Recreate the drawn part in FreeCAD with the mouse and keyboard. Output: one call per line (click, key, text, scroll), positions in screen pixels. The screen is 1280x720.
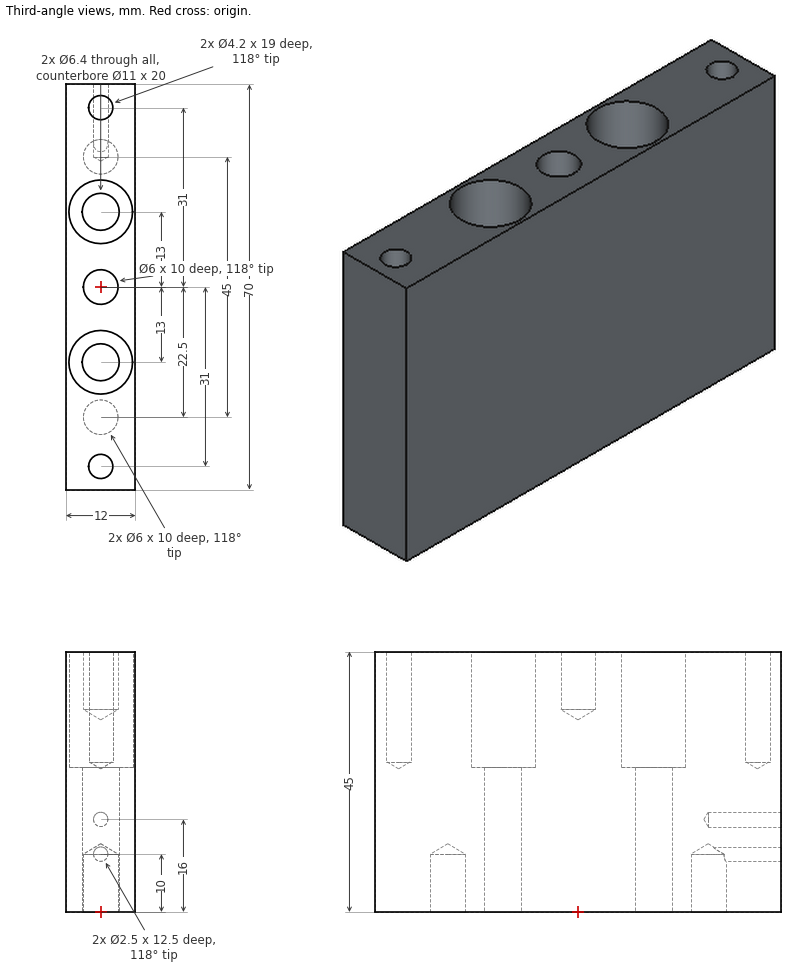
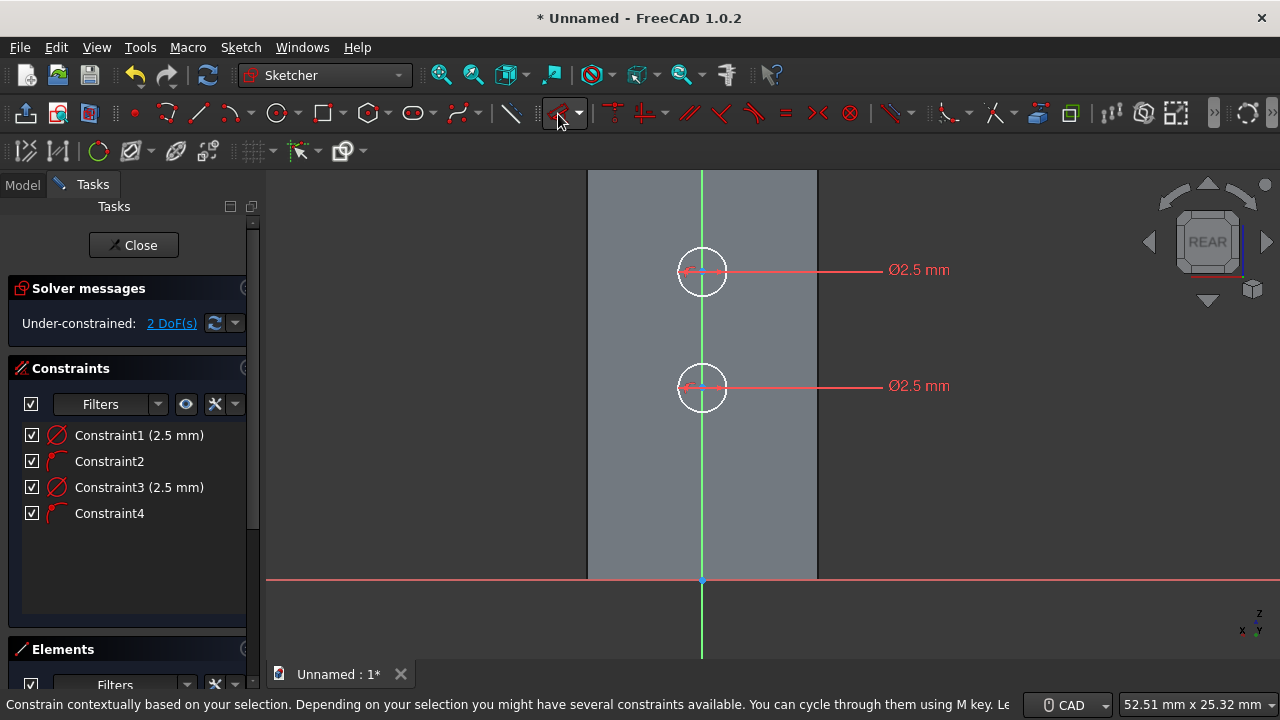
click(702, 388)
click(736, 484)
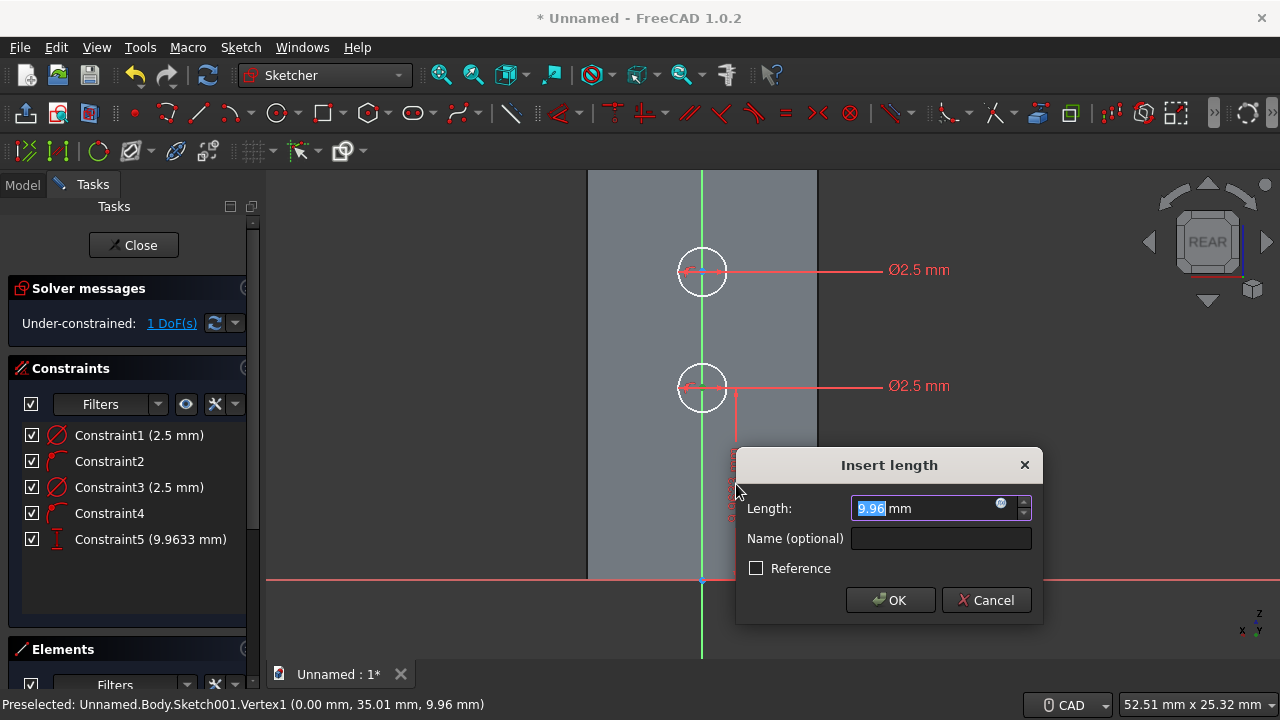
text(10)
key(Return)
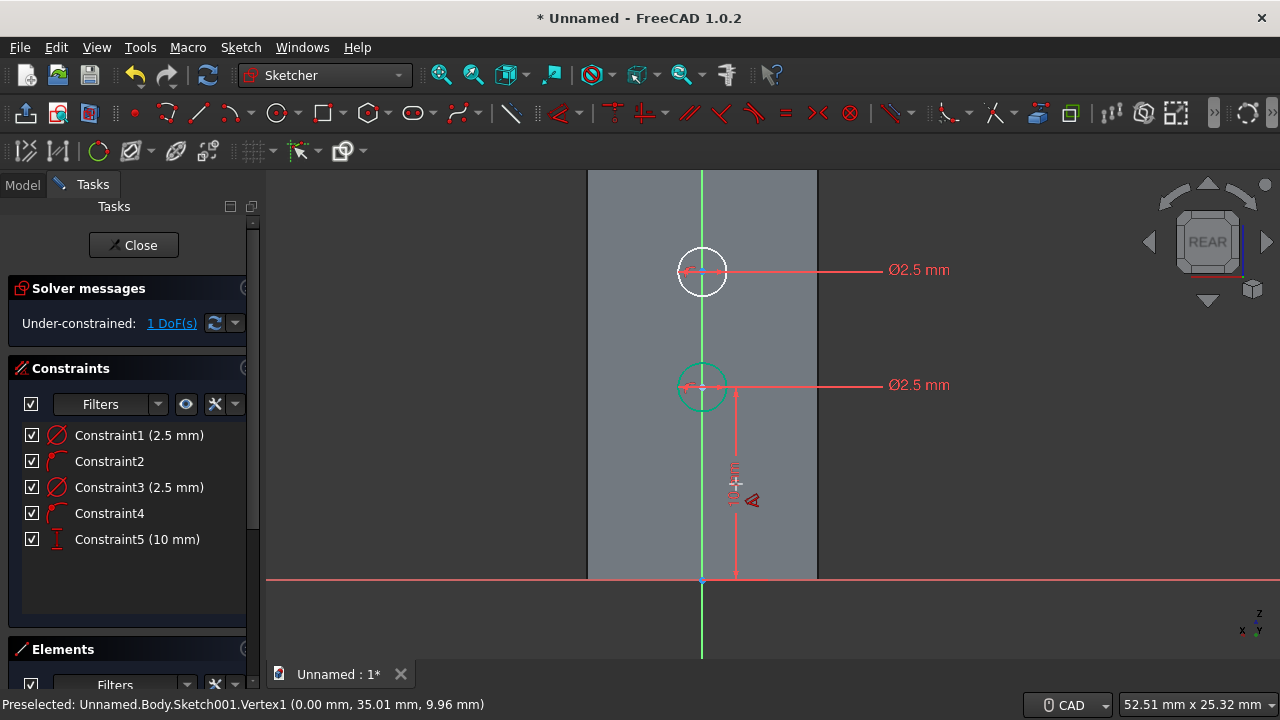
click(702, 272)
click(736, 426)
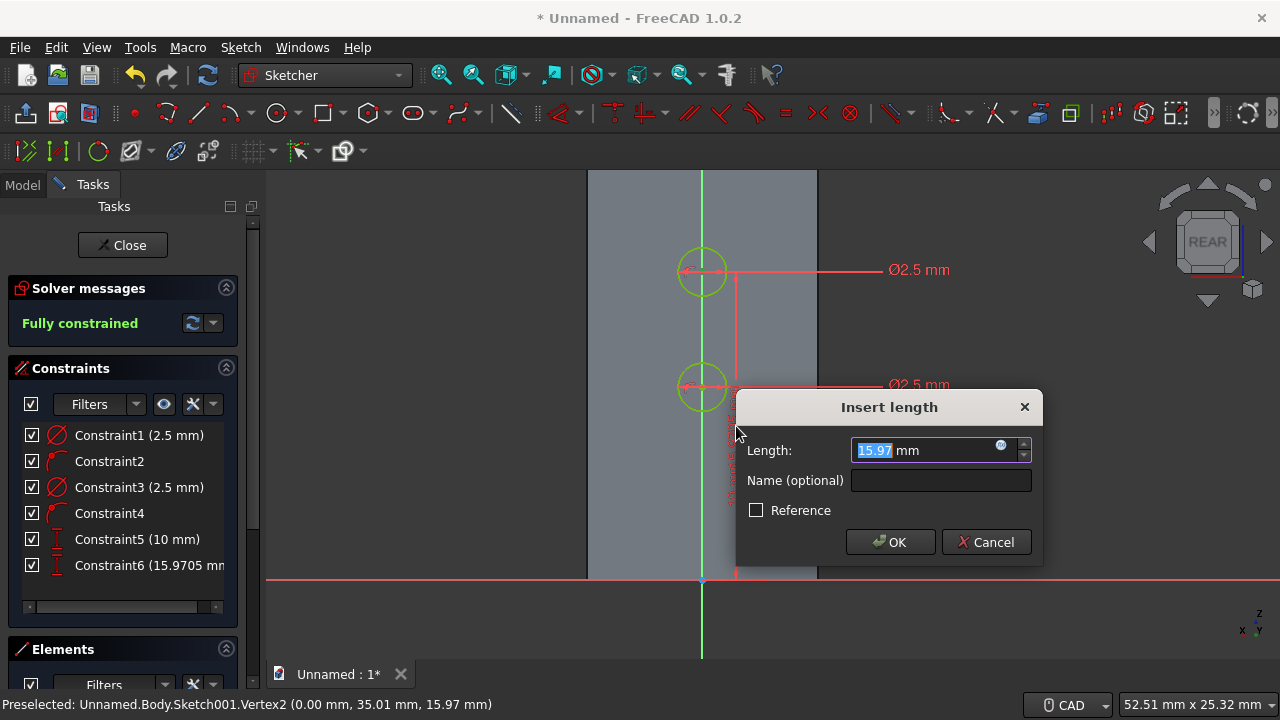
text(16)
key(Return)
key(Escape)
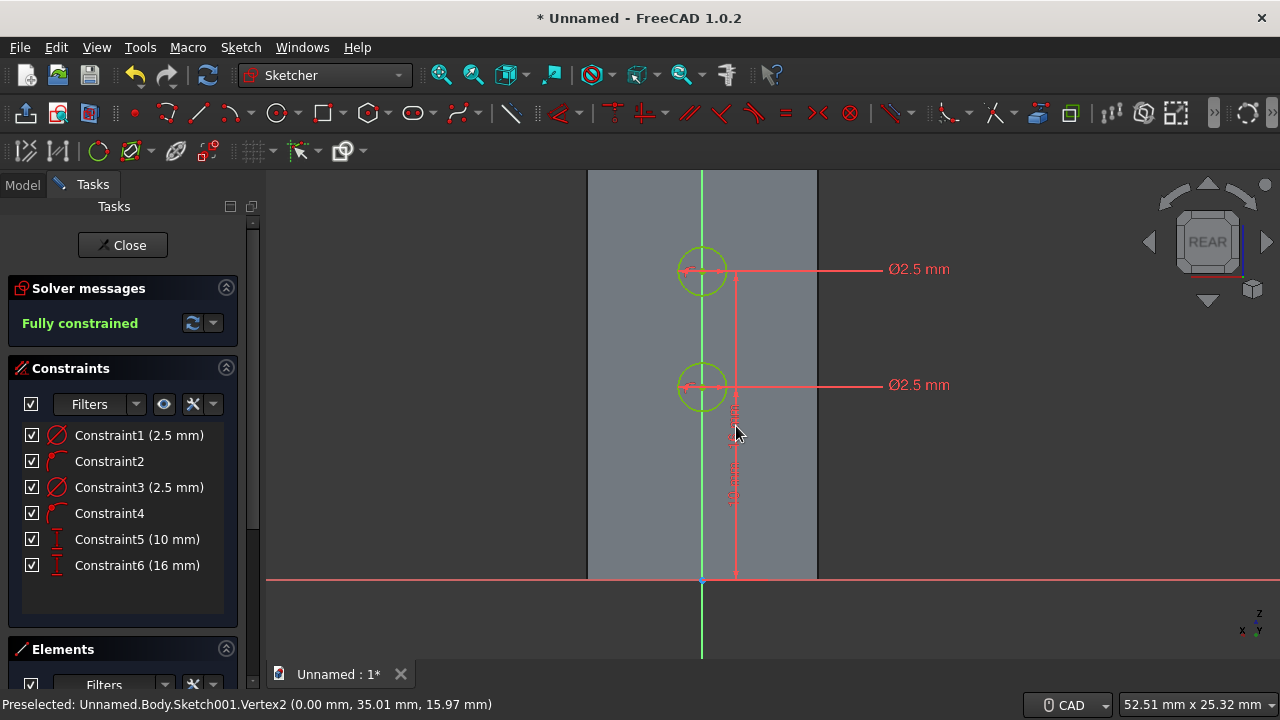
click(123, 245)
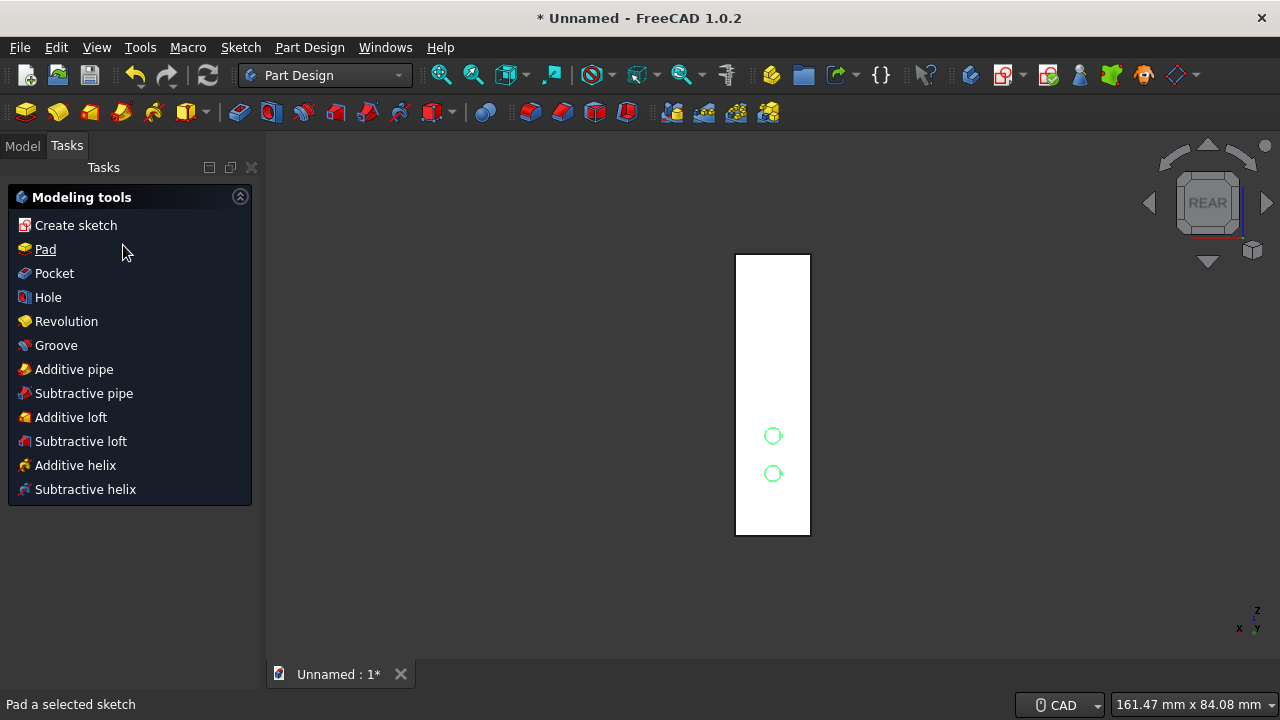
click(272, 112)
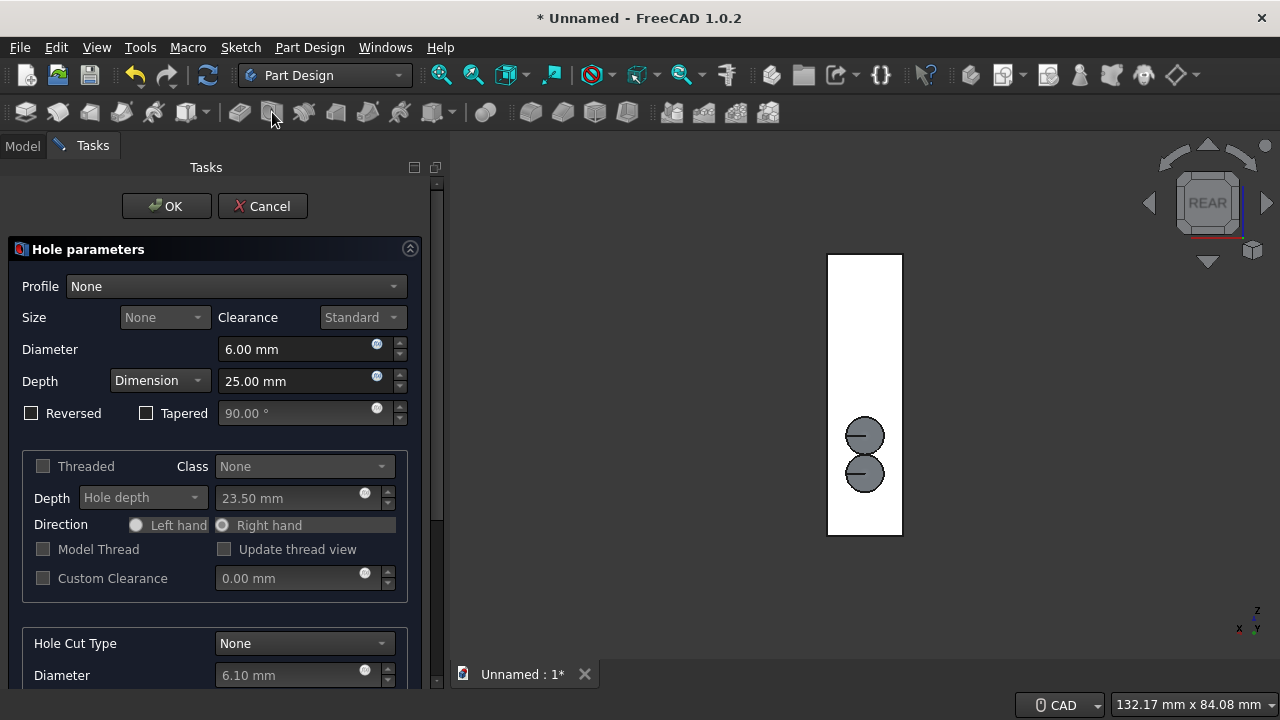
triple_click(305, 349)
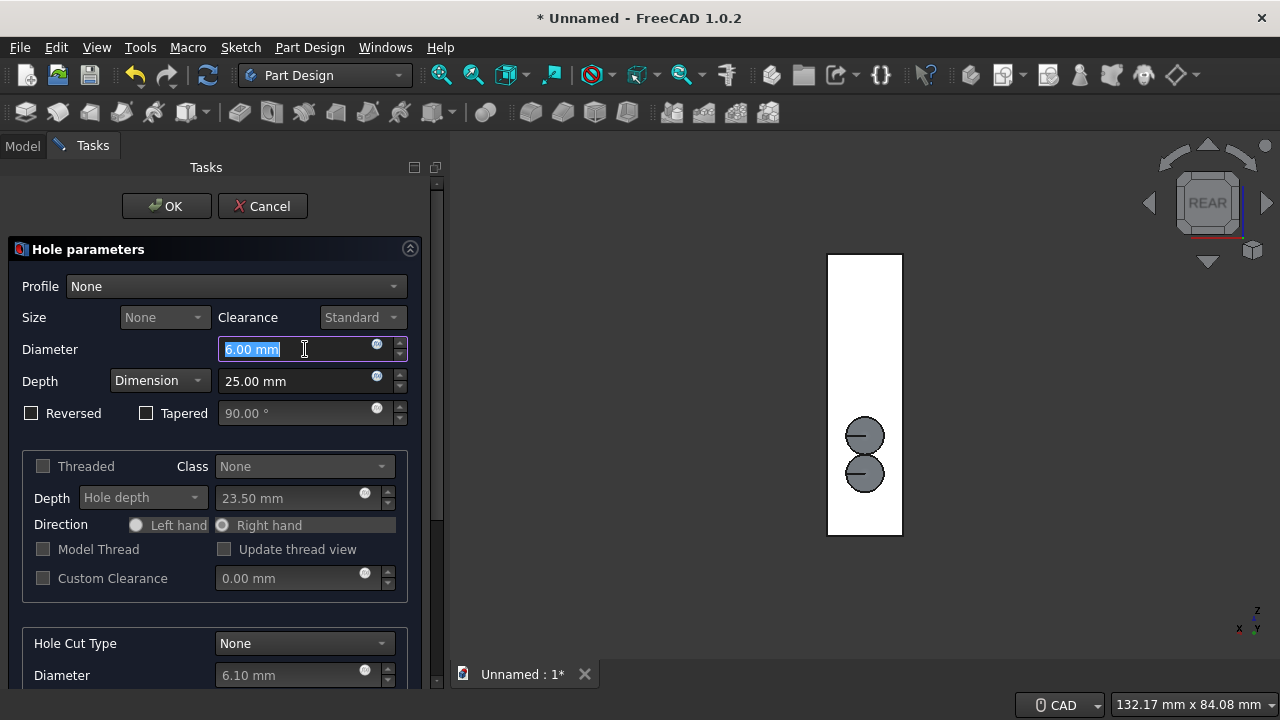
text(2.5)
key(Tab)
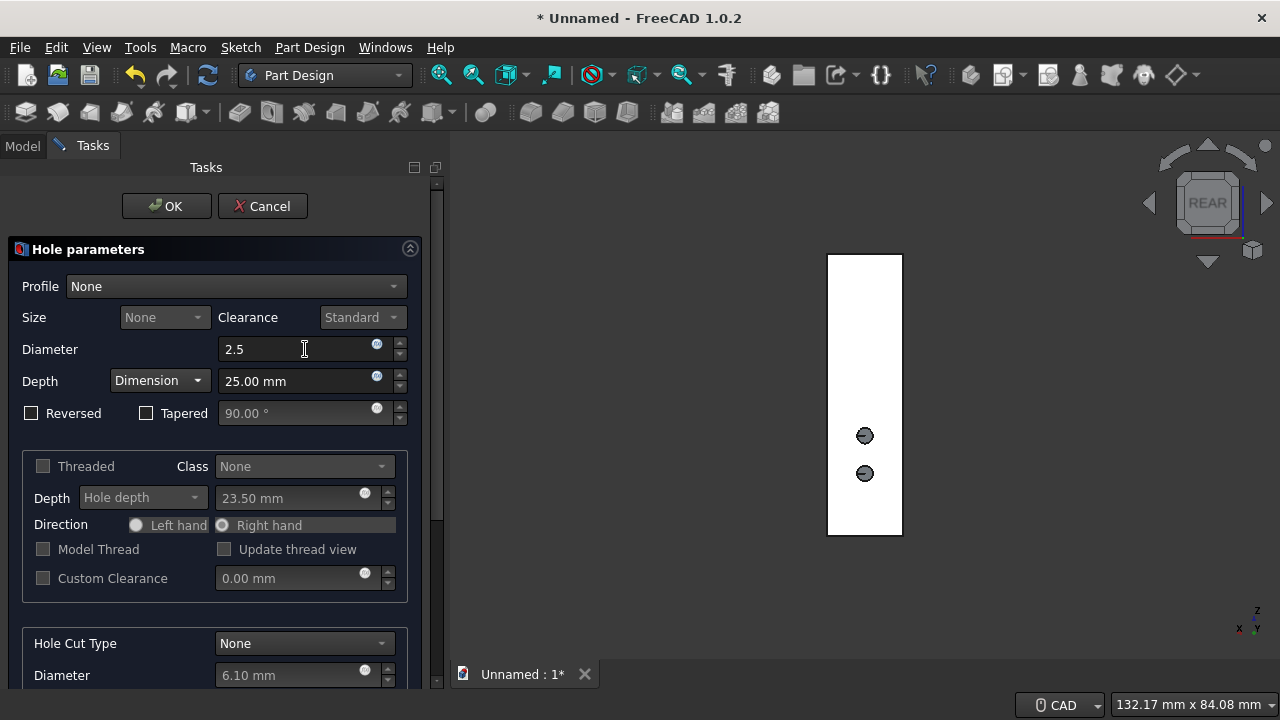
triple_click(305, 381)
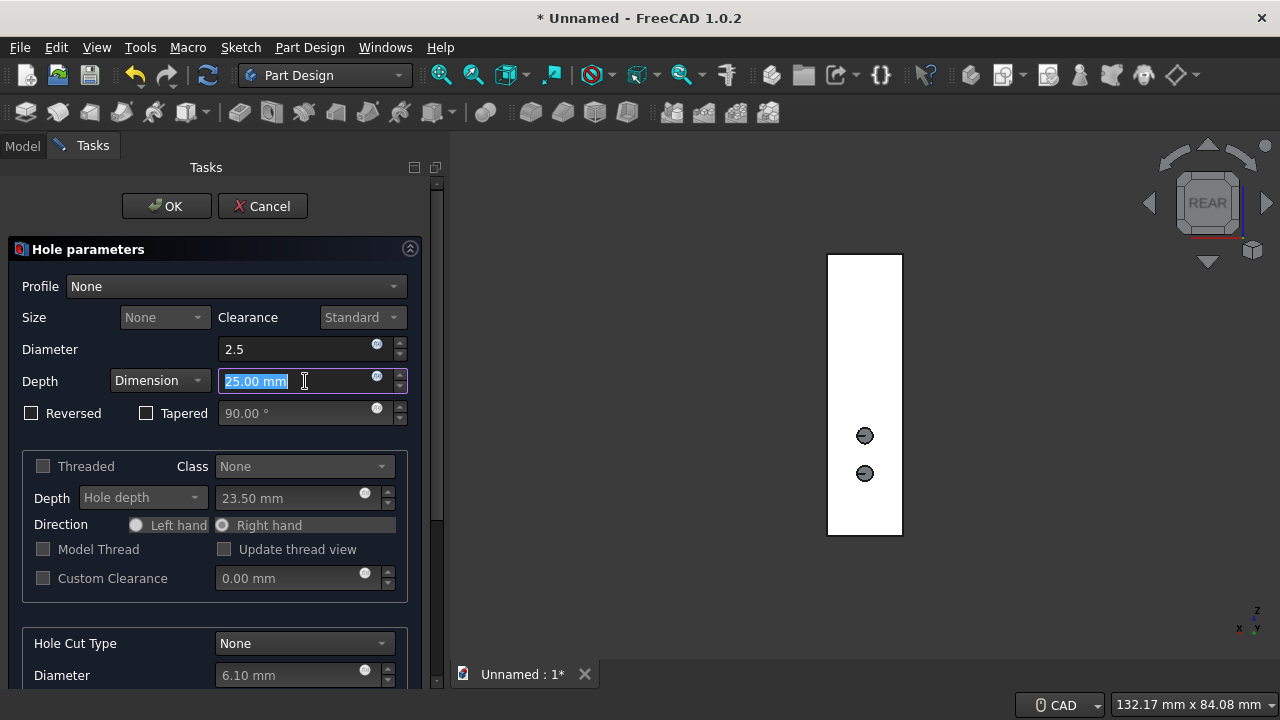
text(12.5)
key(Tab)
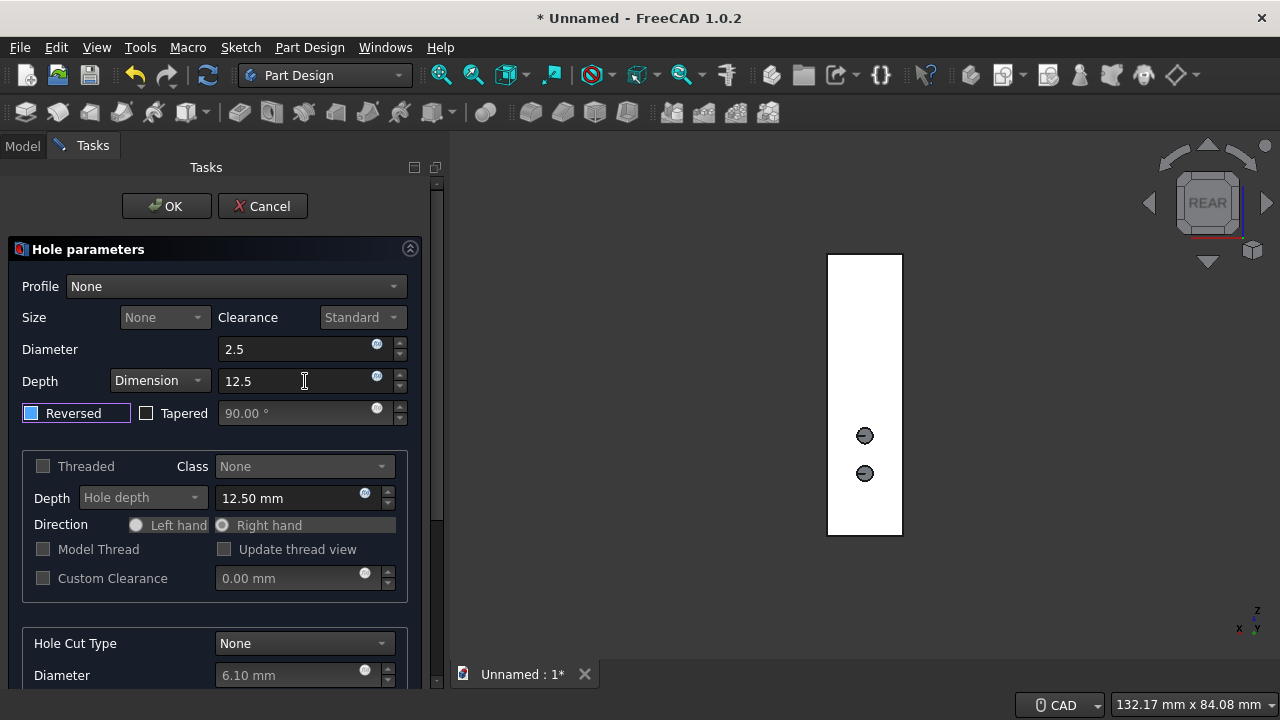
click(167, 206)